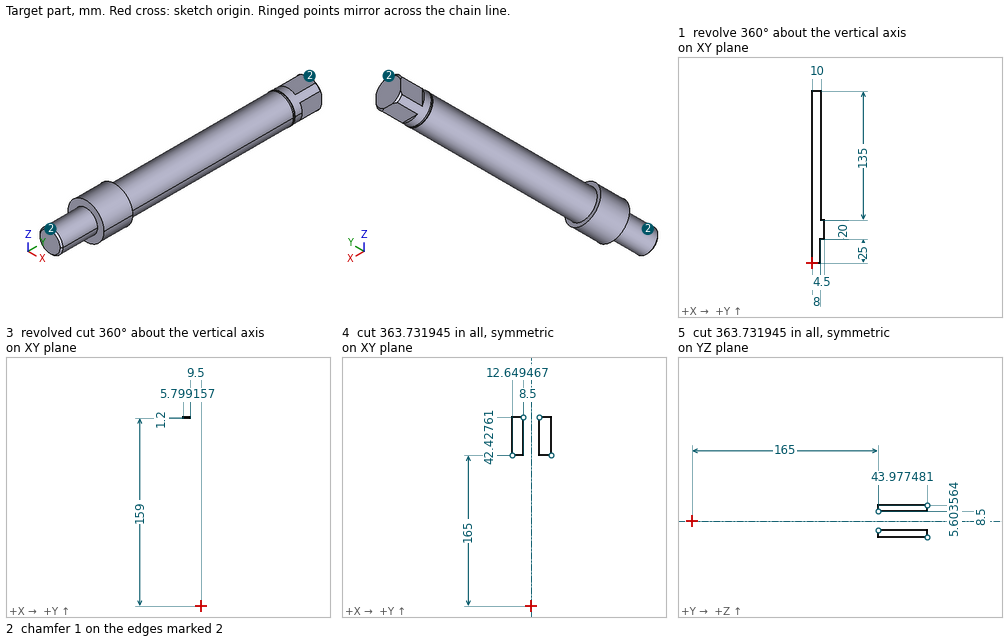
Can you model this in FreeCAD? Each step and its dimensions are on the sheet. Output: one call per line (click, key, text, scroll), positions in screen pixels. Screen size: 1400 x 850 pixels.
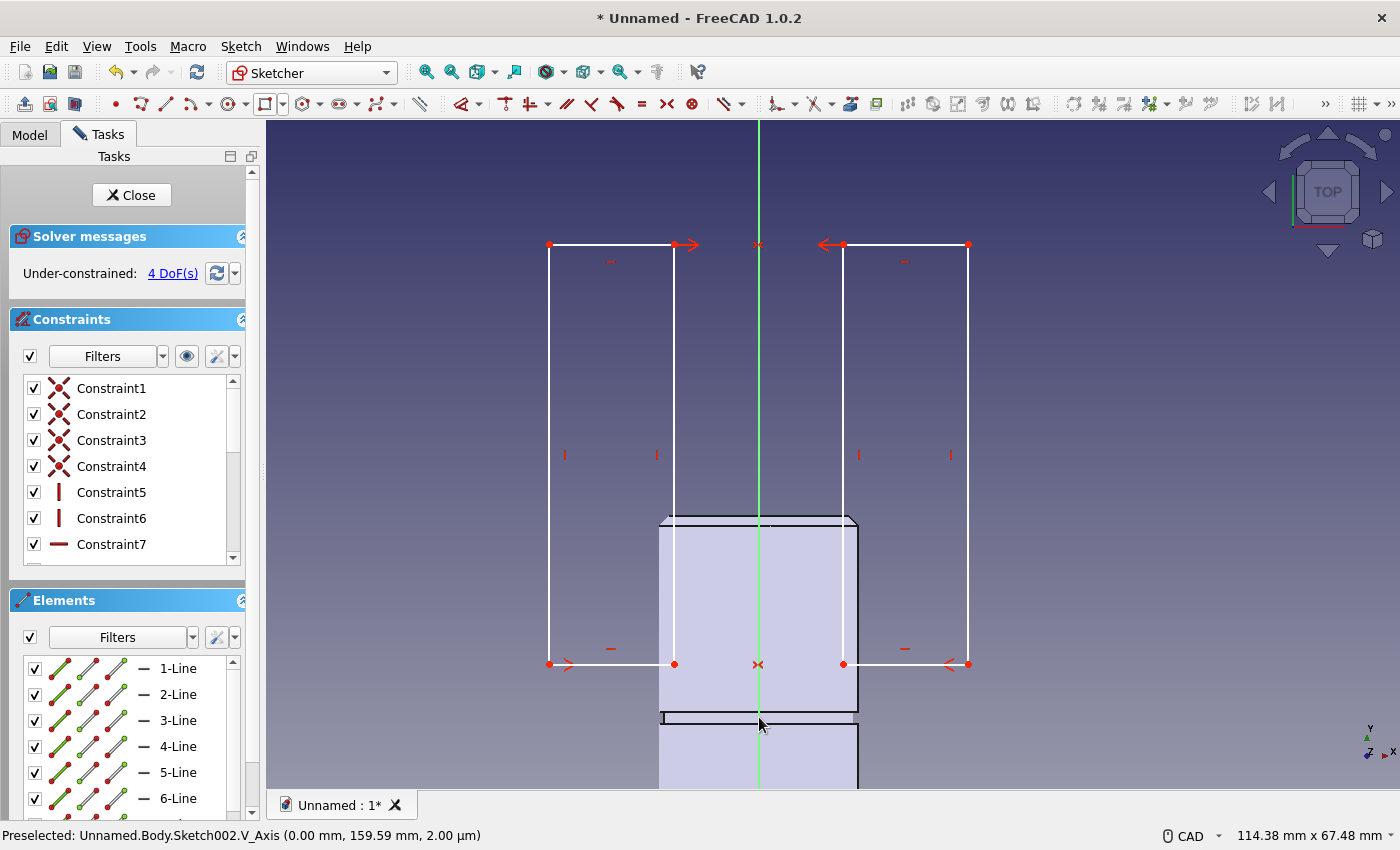
key(d)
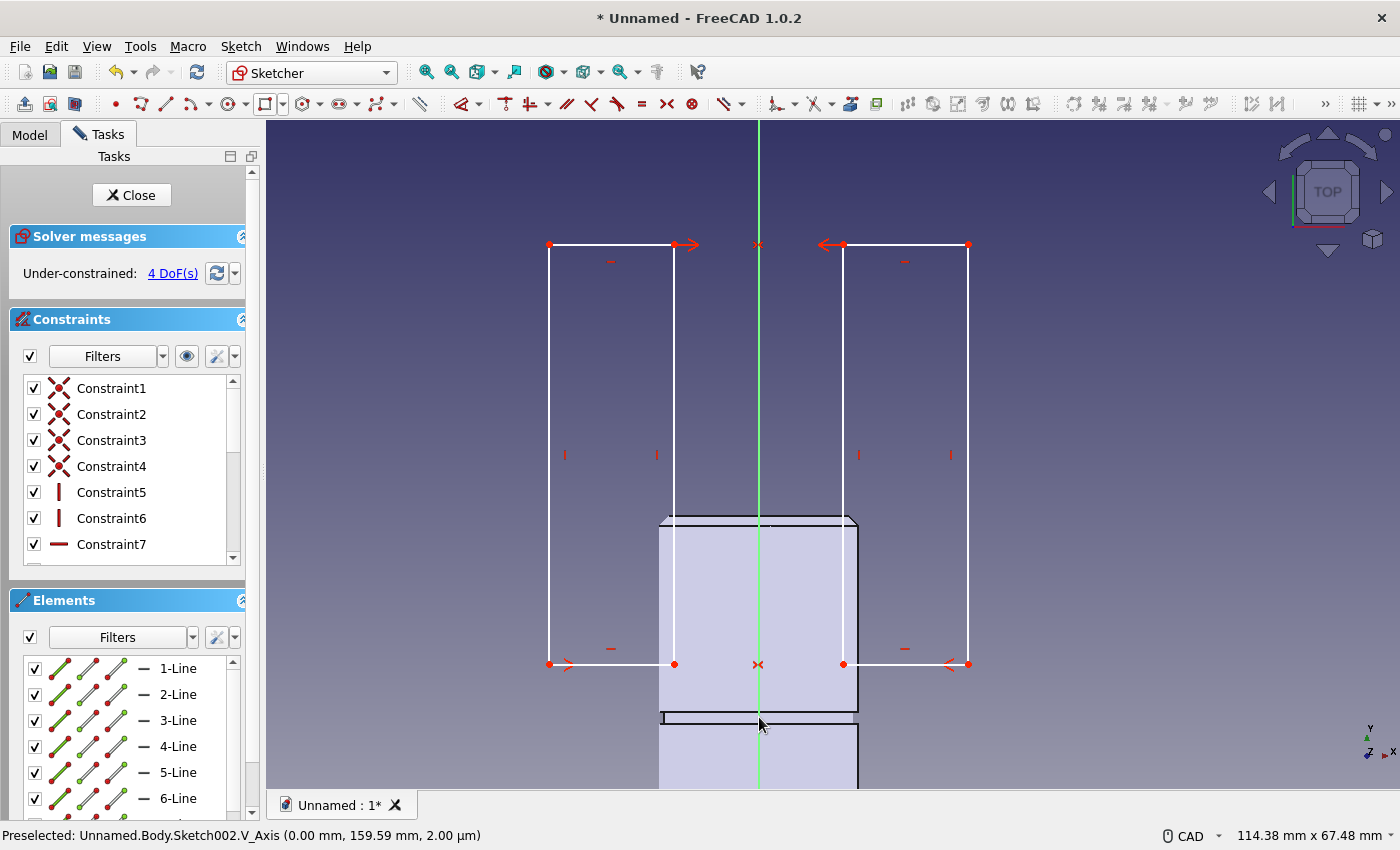
click(549, 665)
click(515, 713)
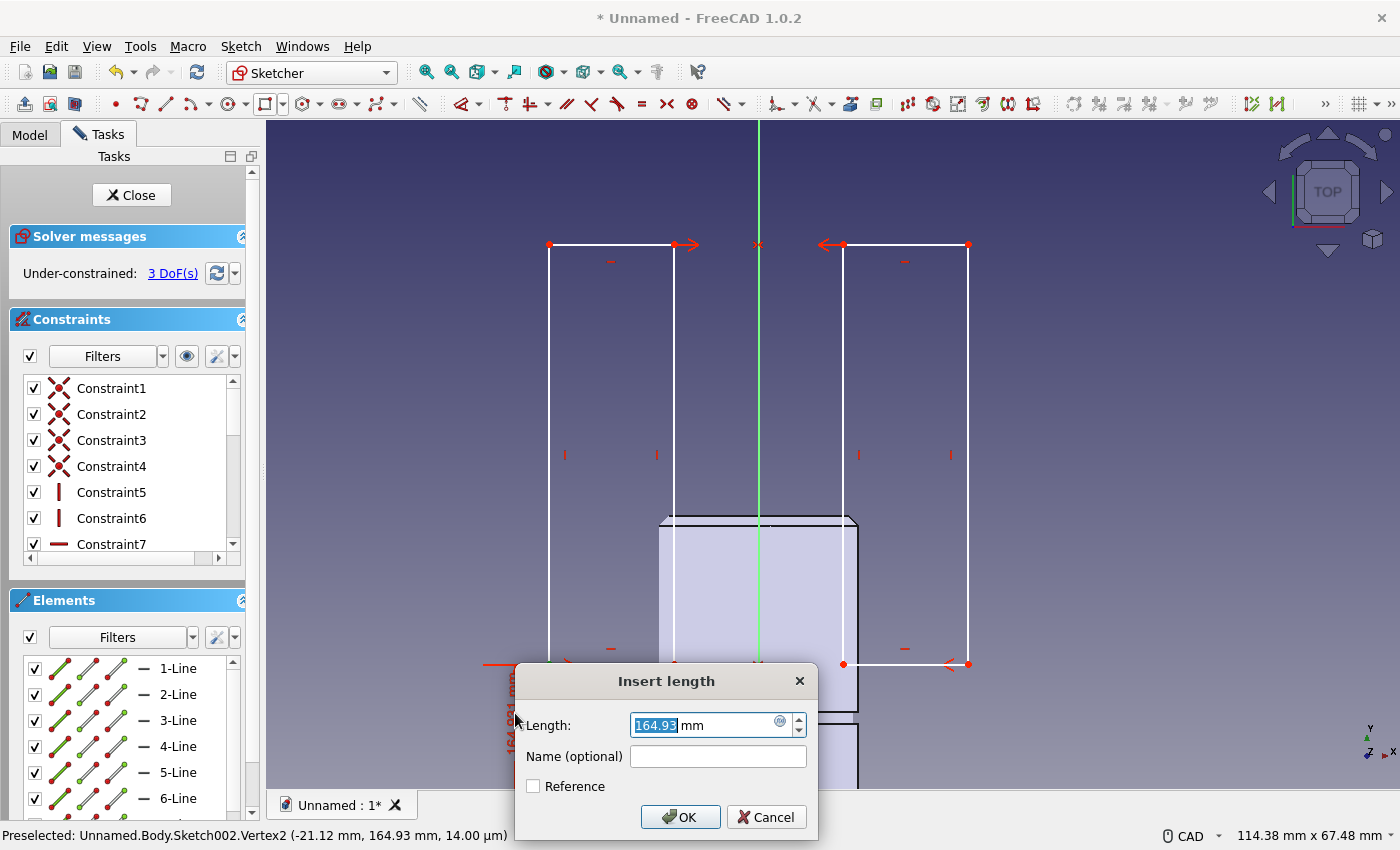
text(165)
key(Return)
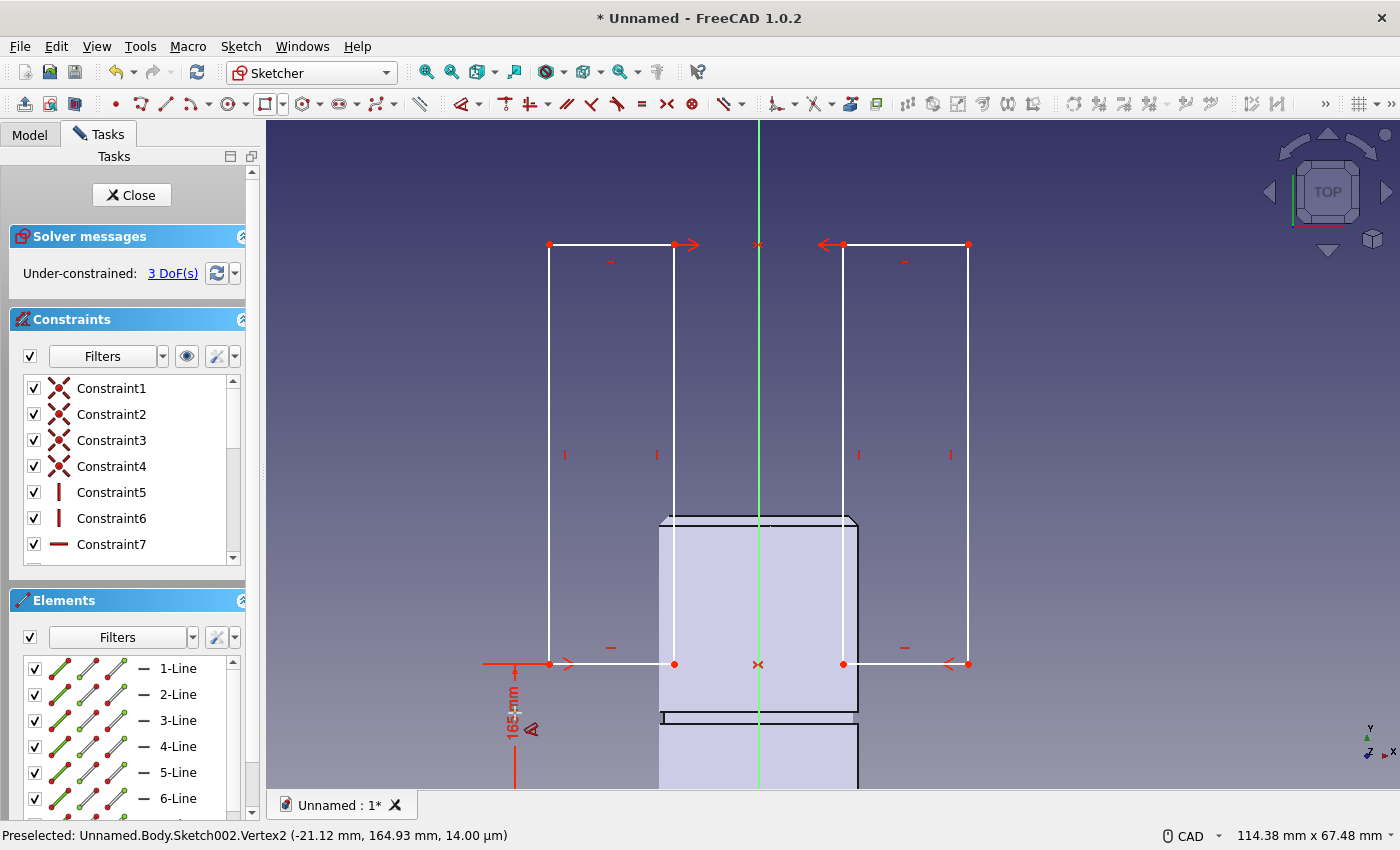
click(674, 664)
click(716, 630)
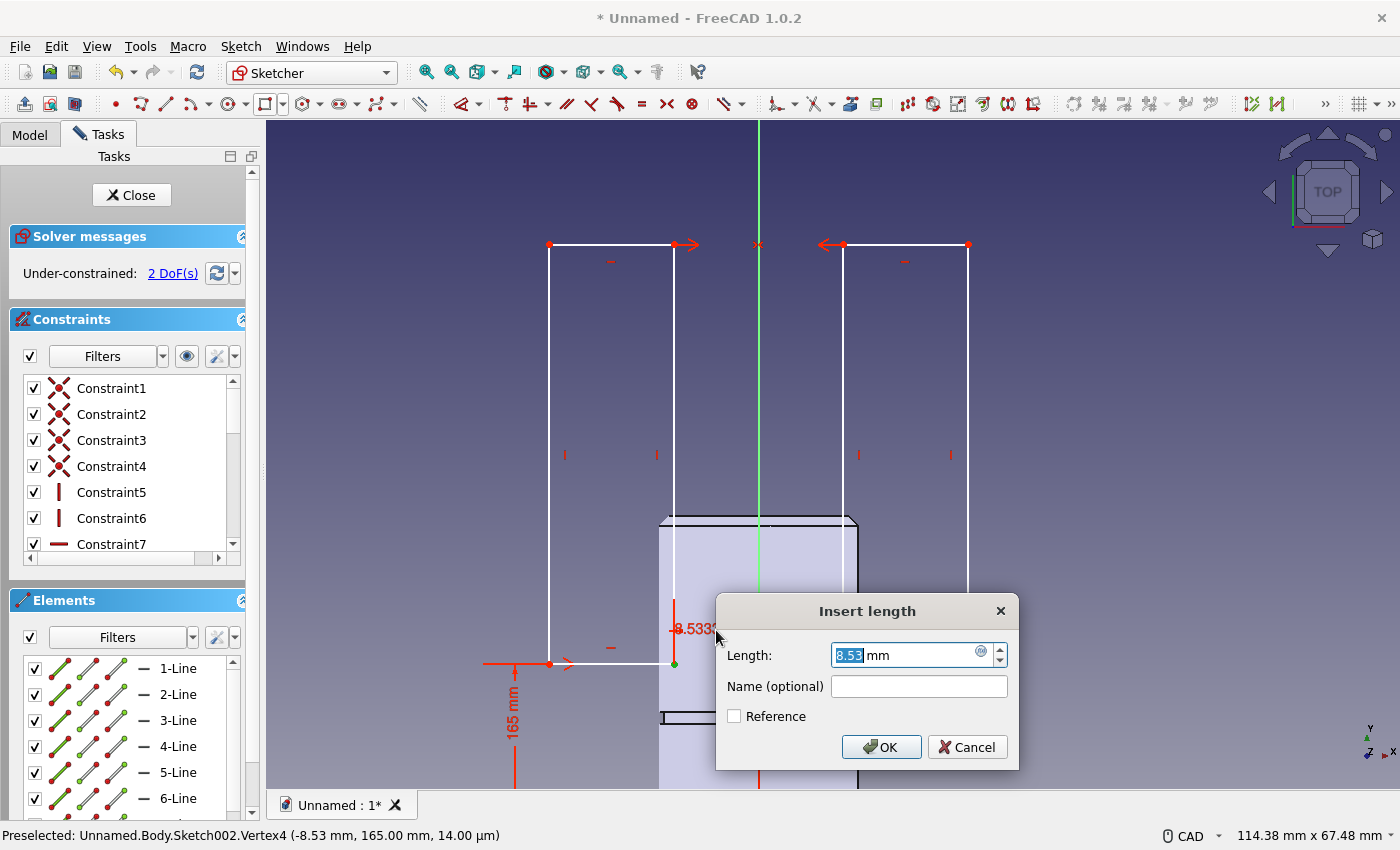
text(8.5)
key(Return)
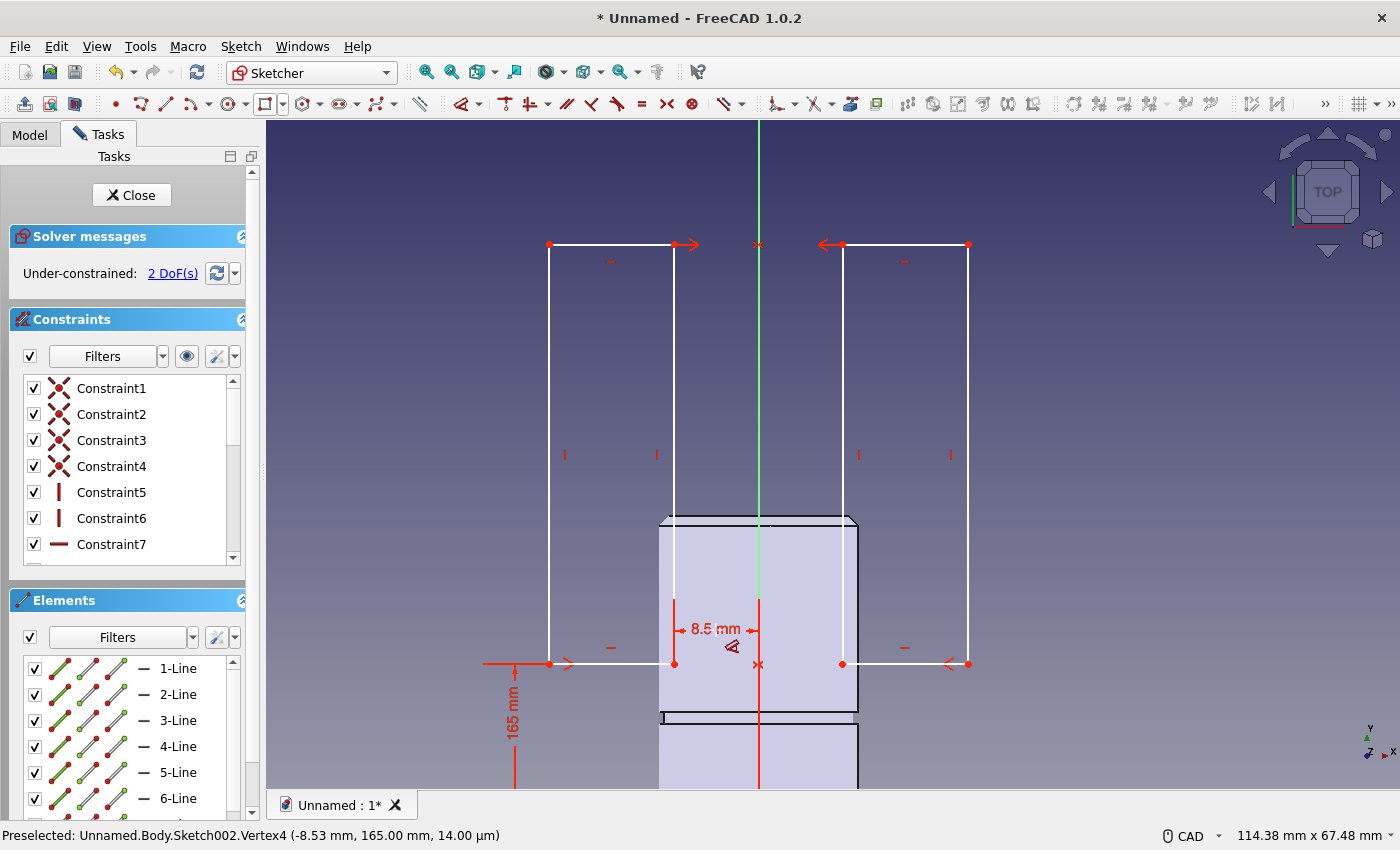
click(549, 371)
click(515, 455)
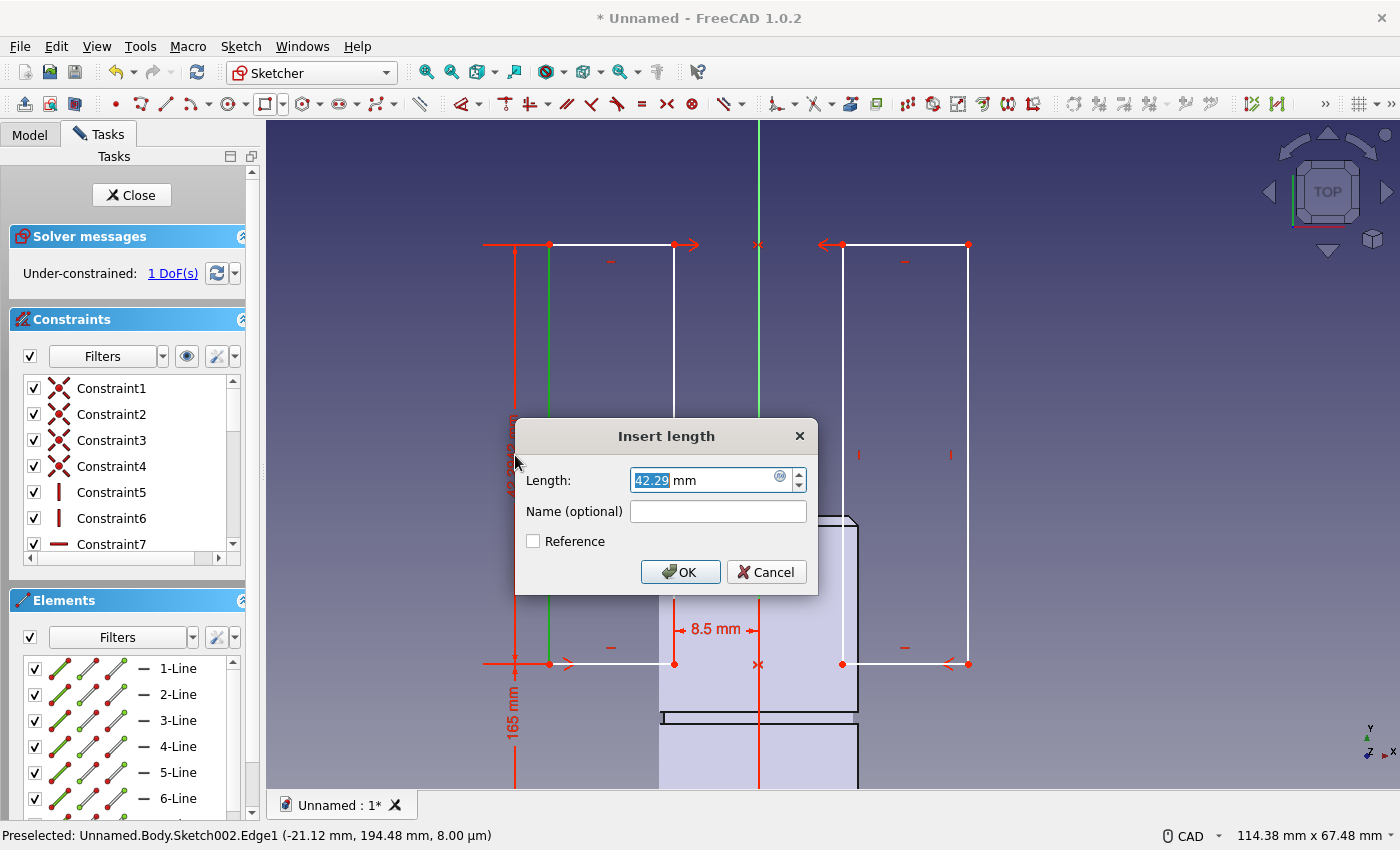
text(42.42761)
key(Return)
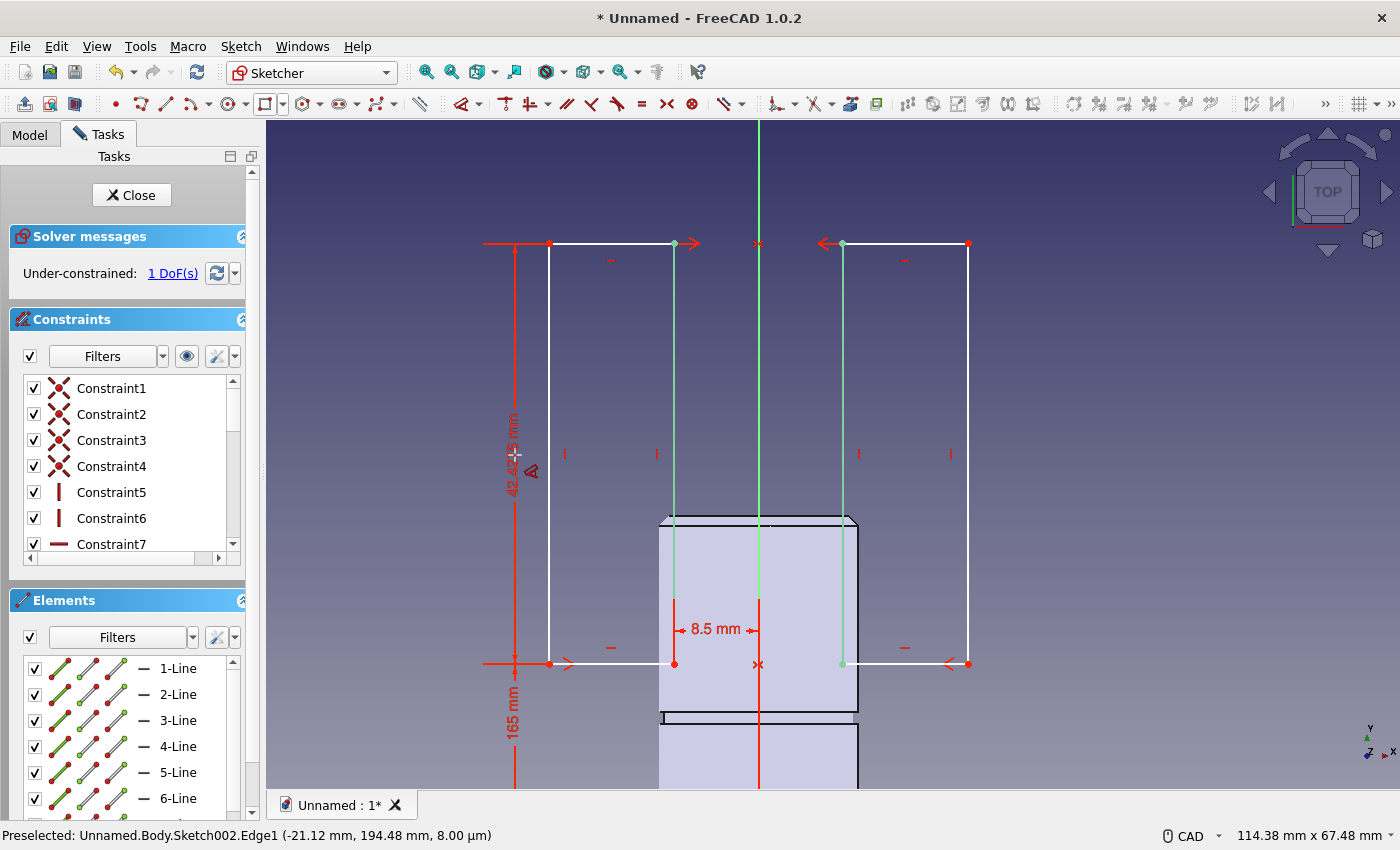
click(587, 664)
click(612, 698)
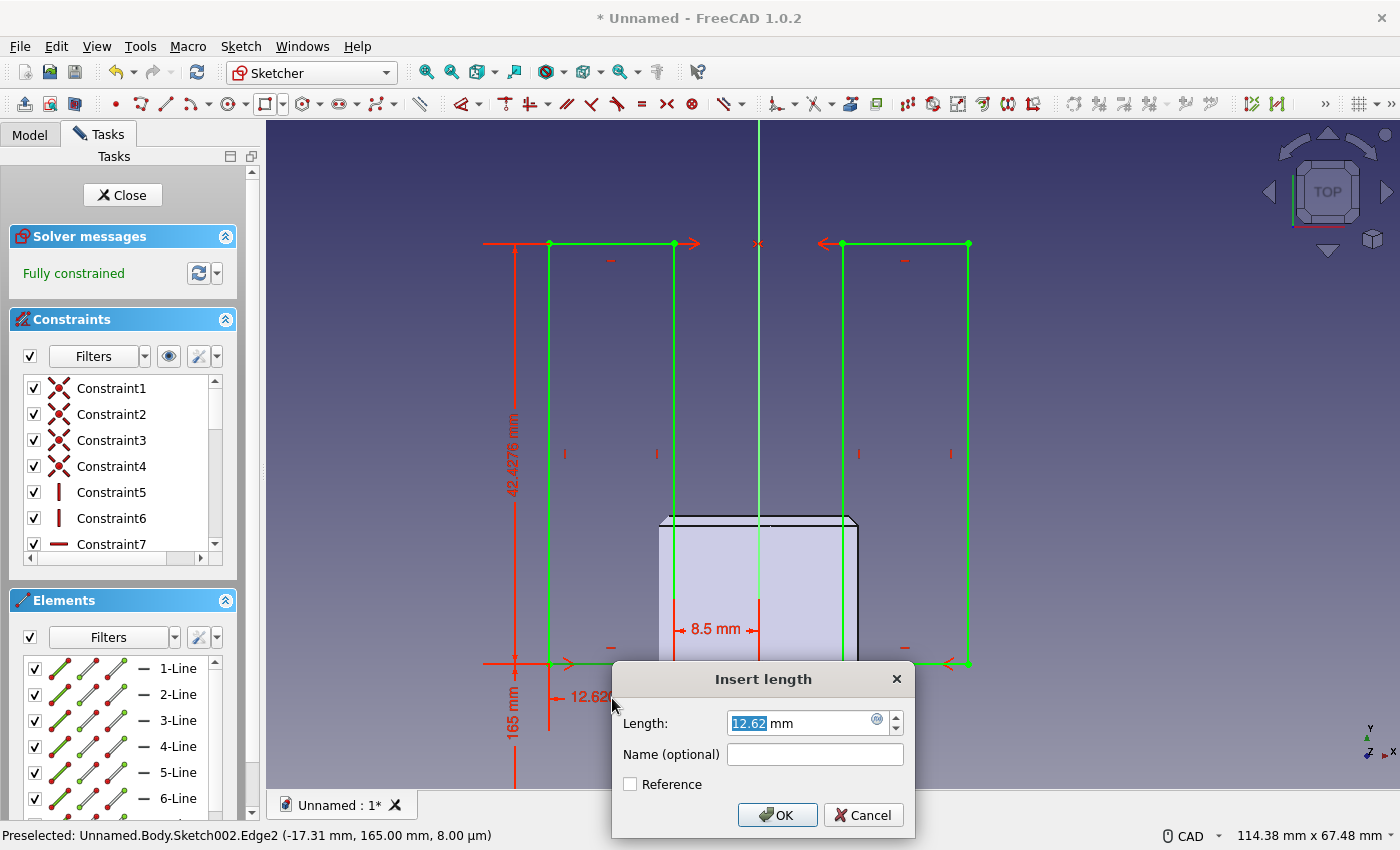
text(12.649467)
key(Return)
key(Escape)